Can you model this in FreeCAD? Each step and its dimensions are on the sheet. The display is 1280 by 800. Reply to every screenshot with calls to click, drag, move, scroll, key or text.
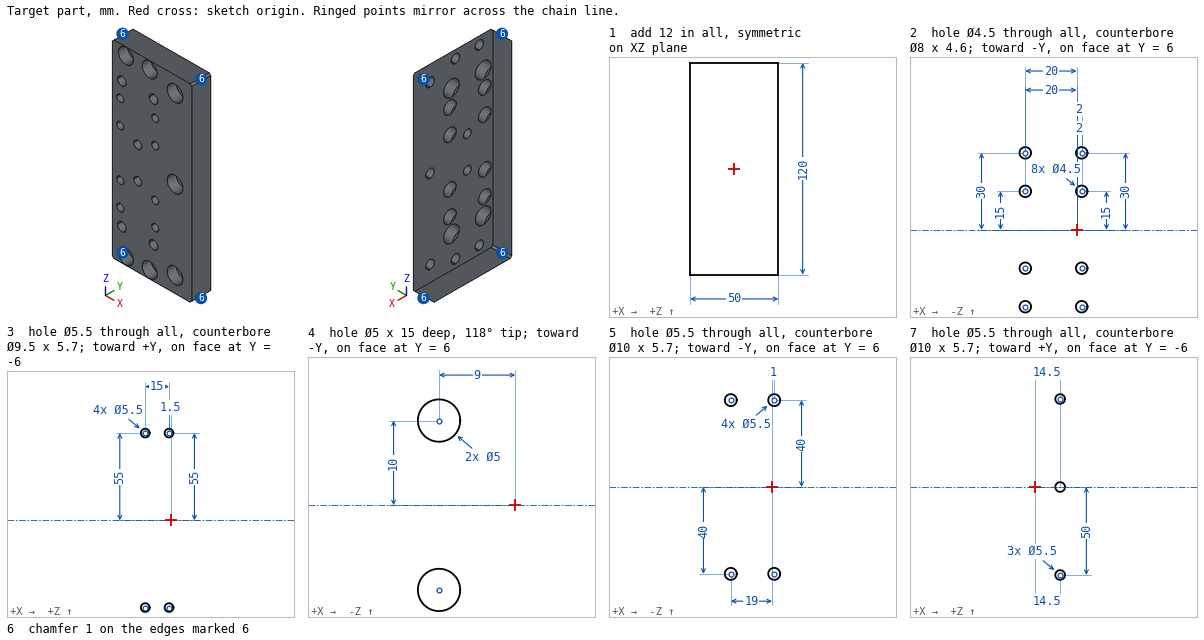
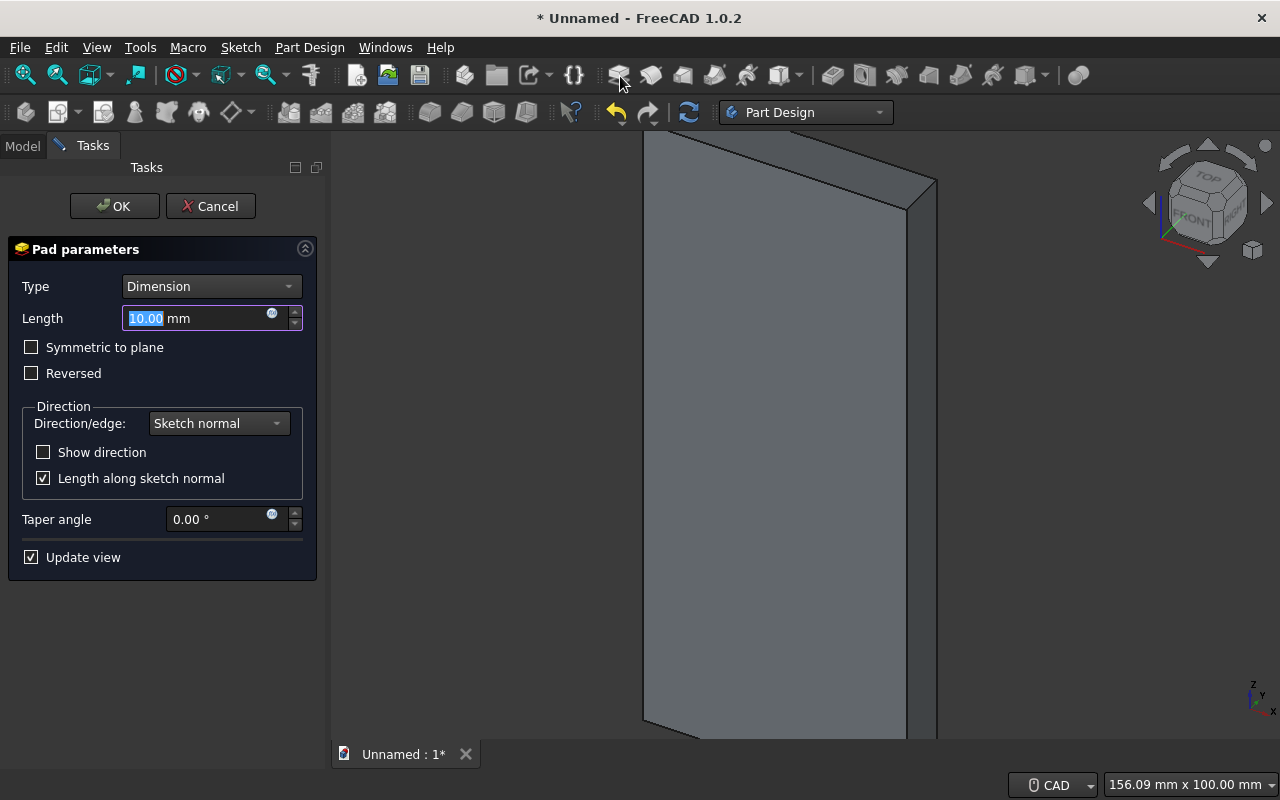
text(12)
key(Tab)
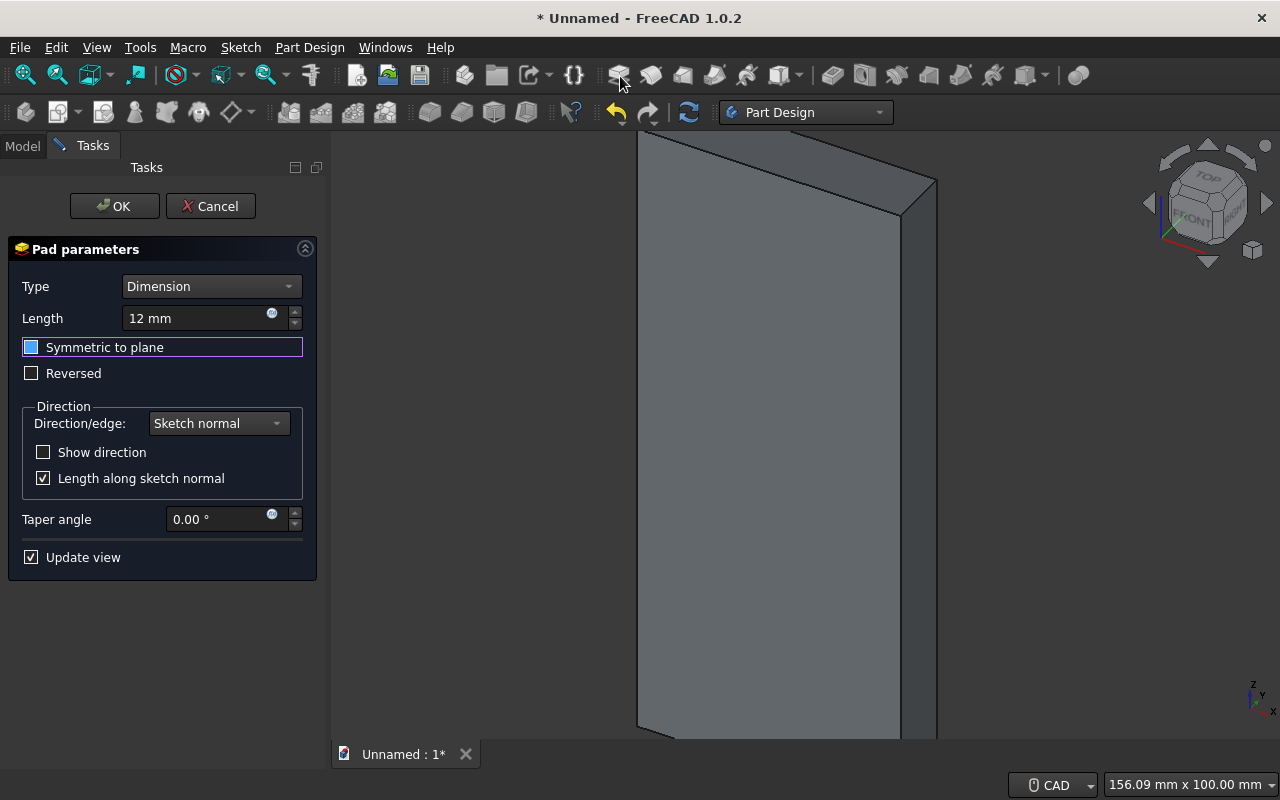
click(30, 347)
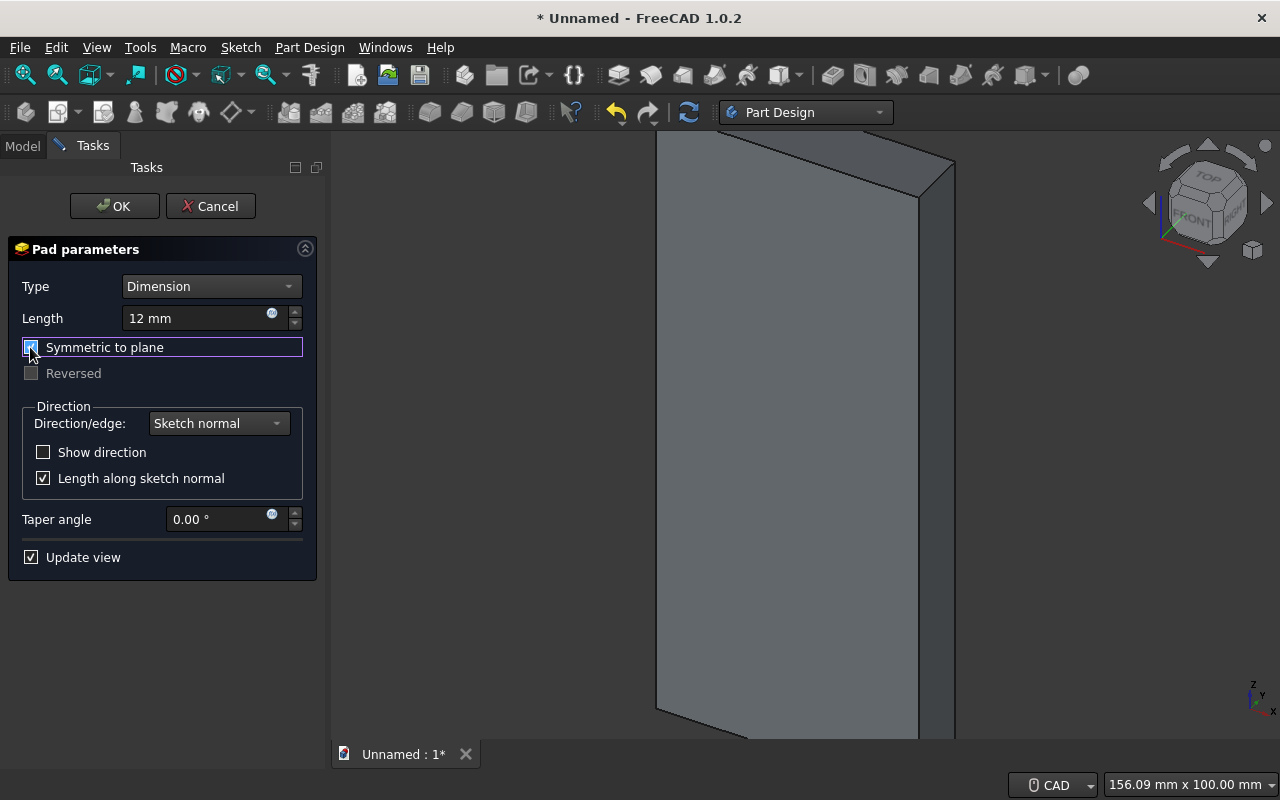
click(115, 206)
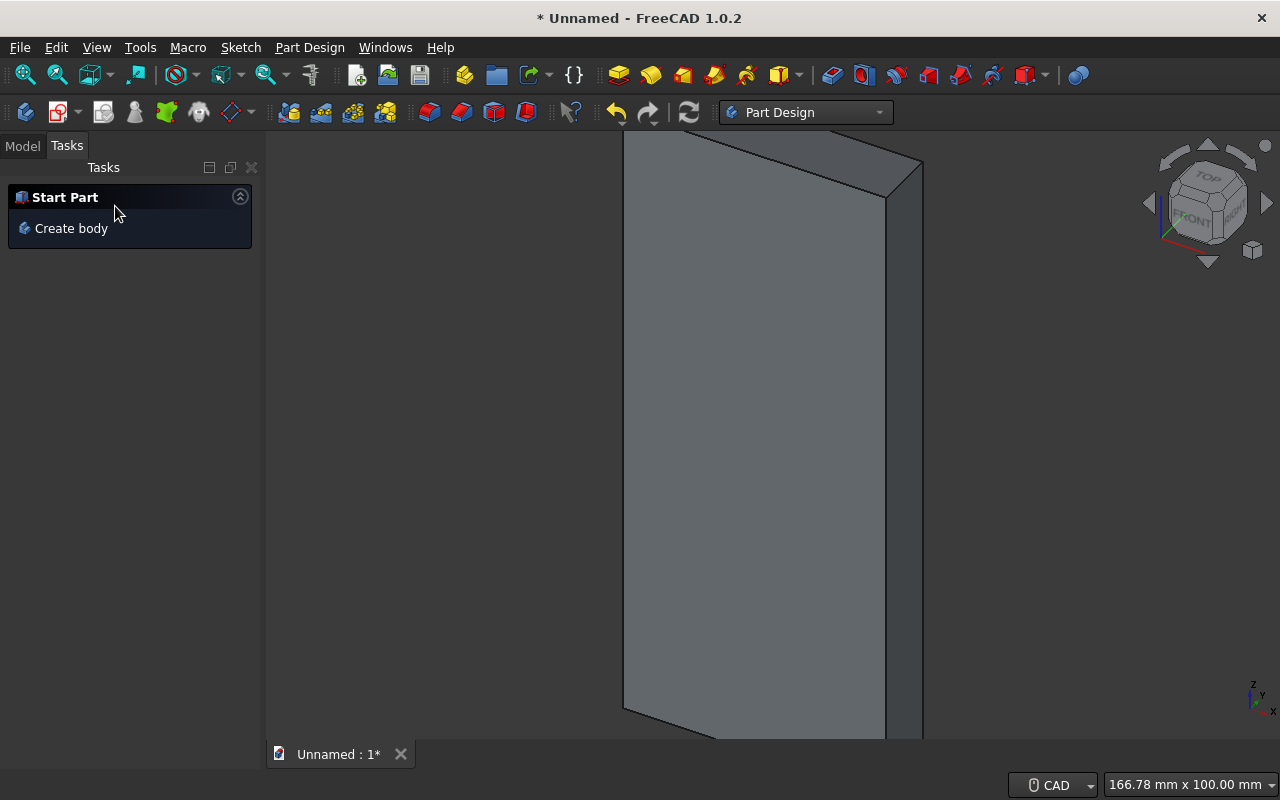
click(26, 76)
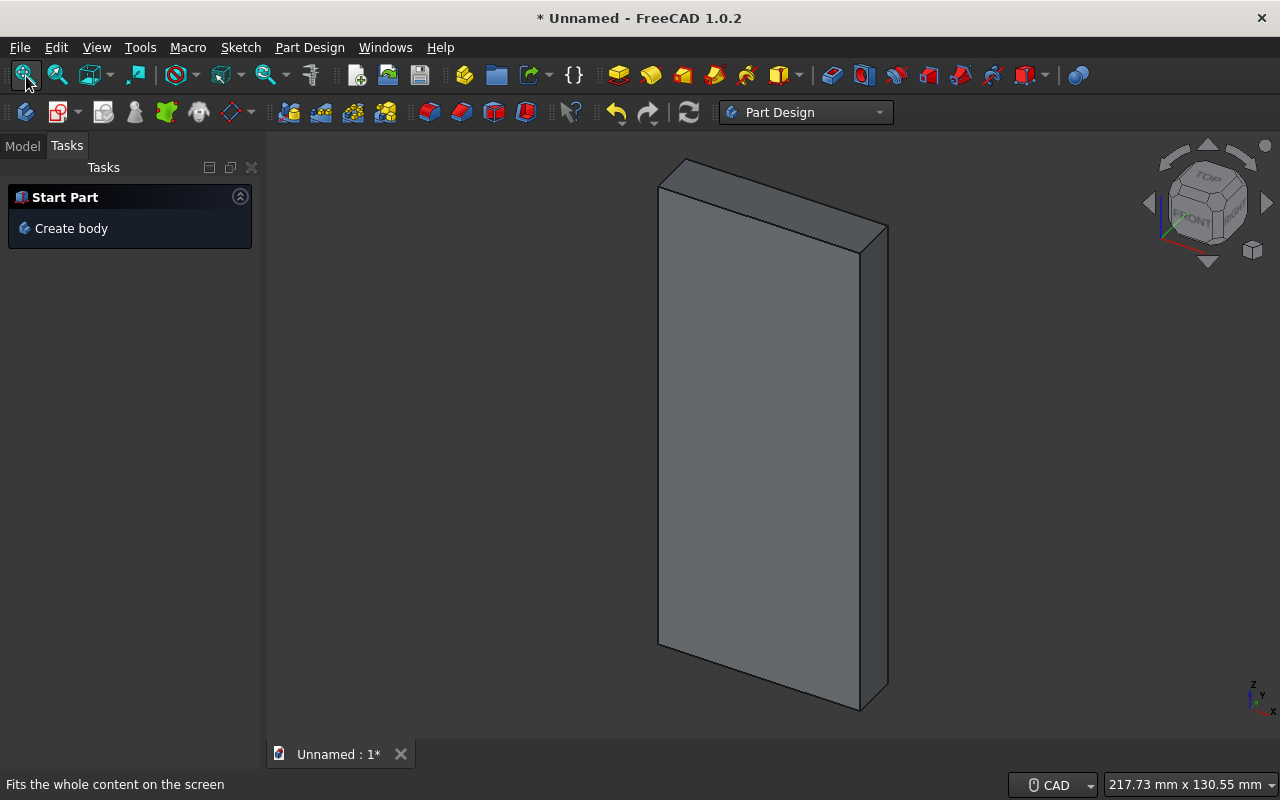
key(4)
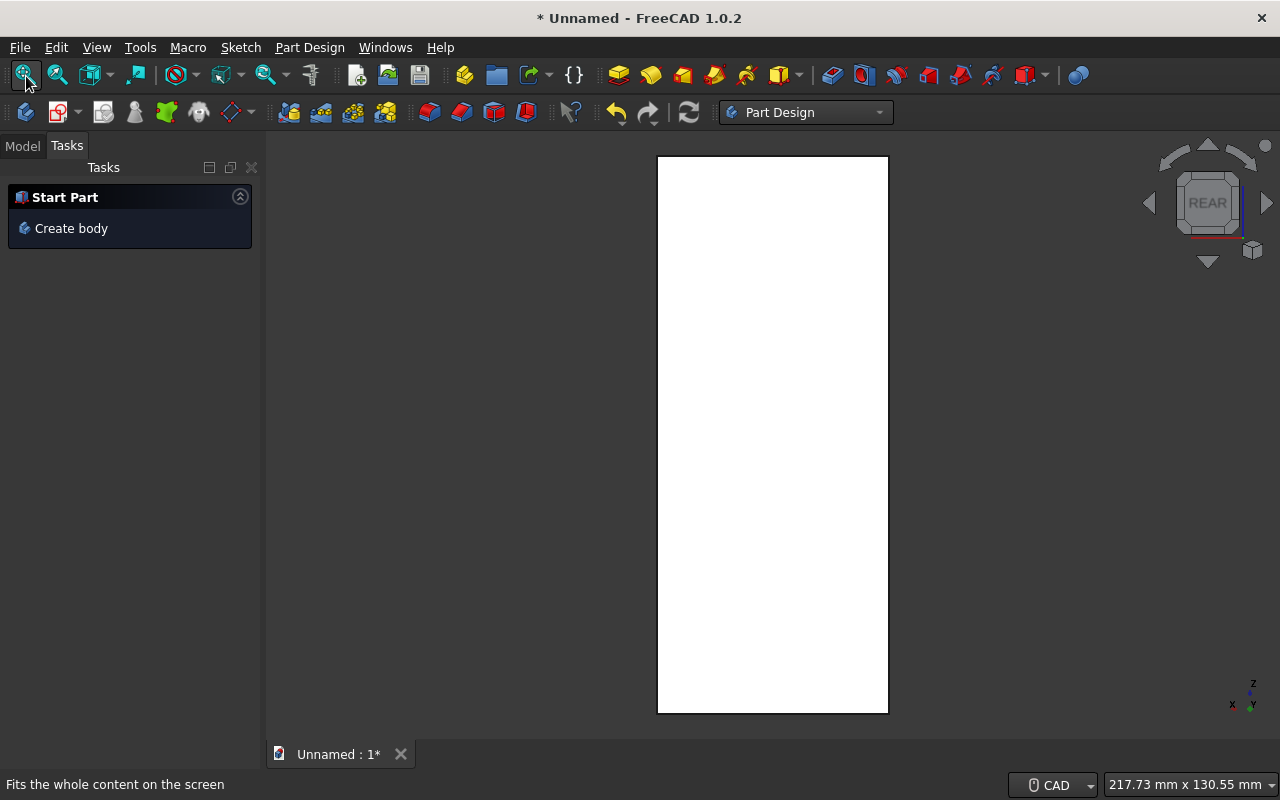
click(773, 274)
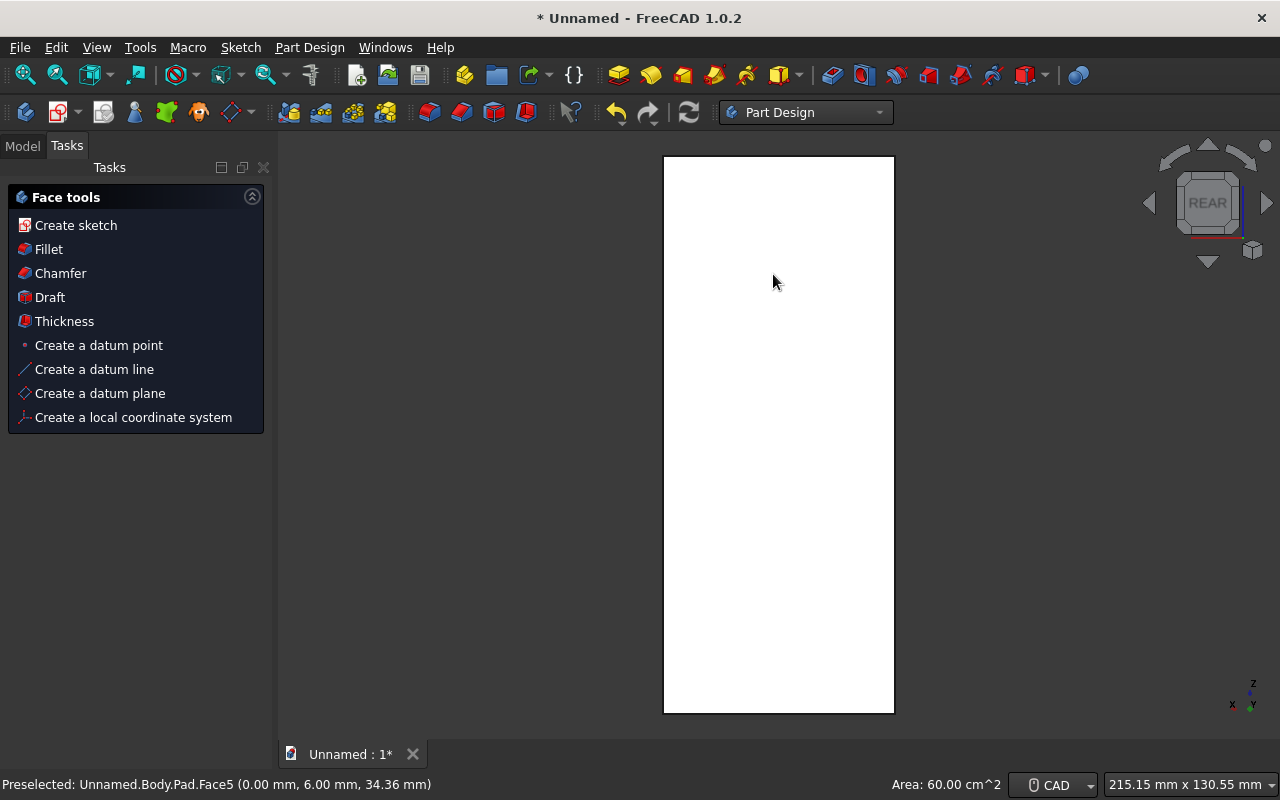
click(58, 112)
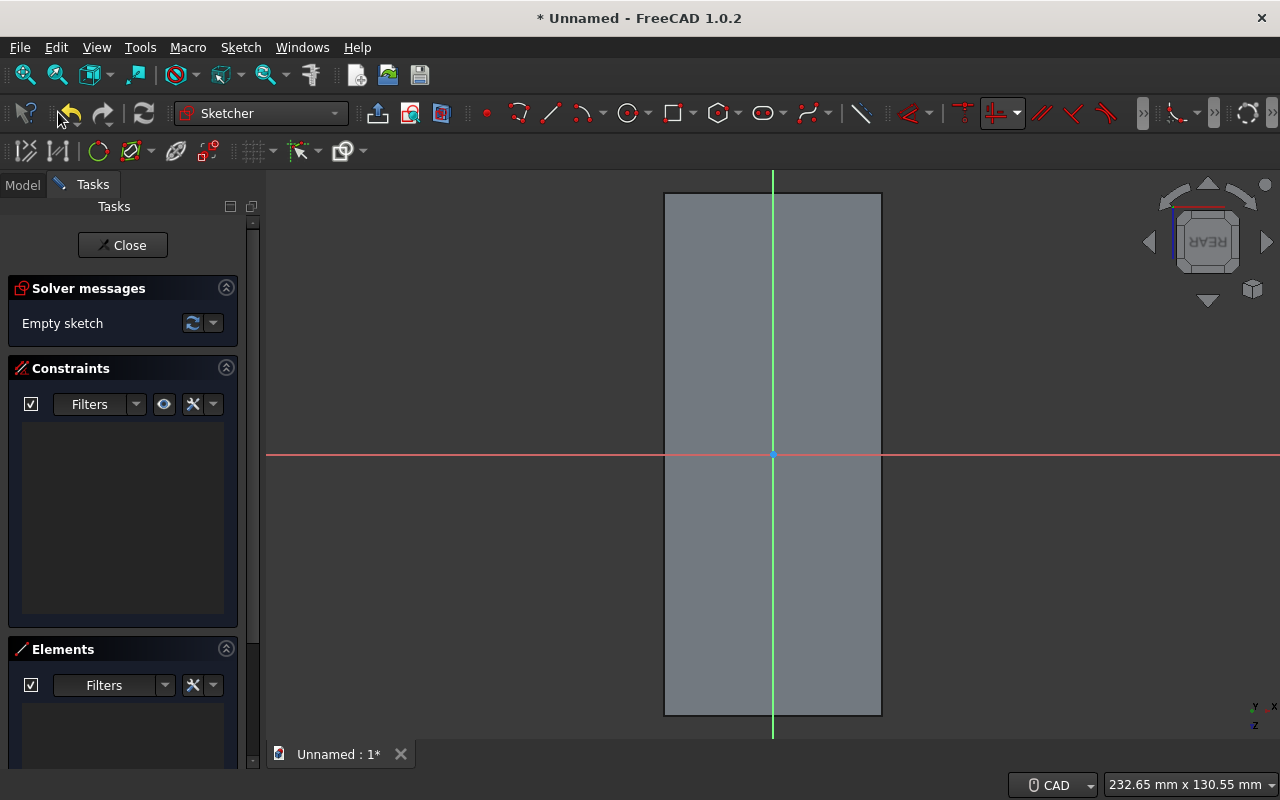
click(628, 114)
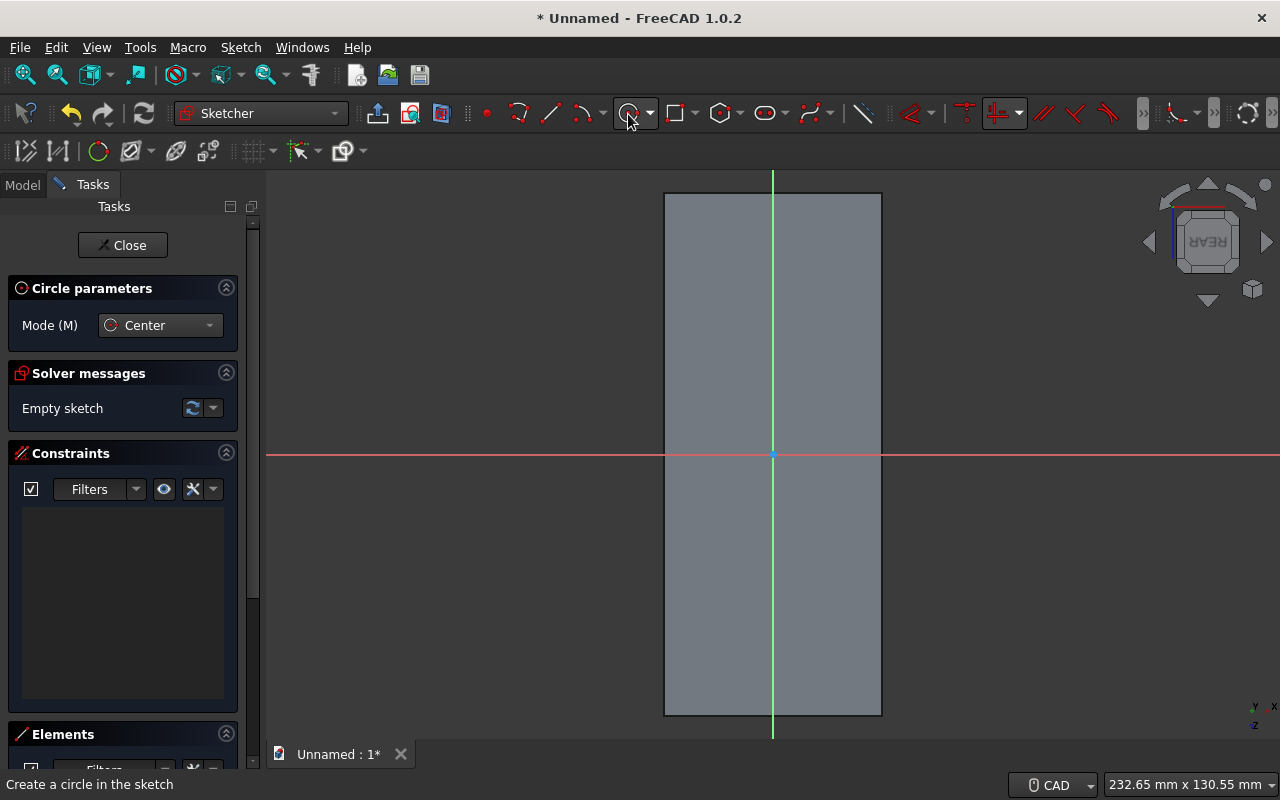
scroll(782, 389, up, 5)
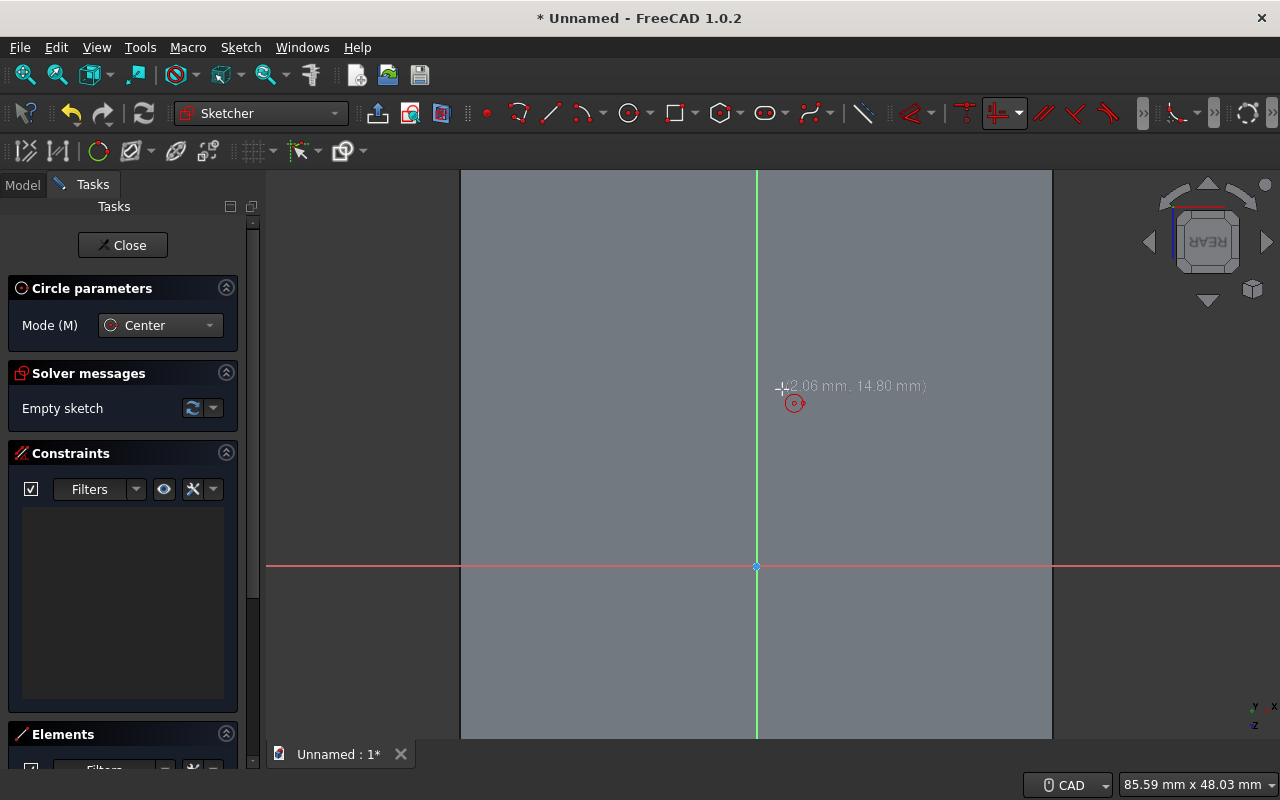
click(780, 389)
move(799, 370)